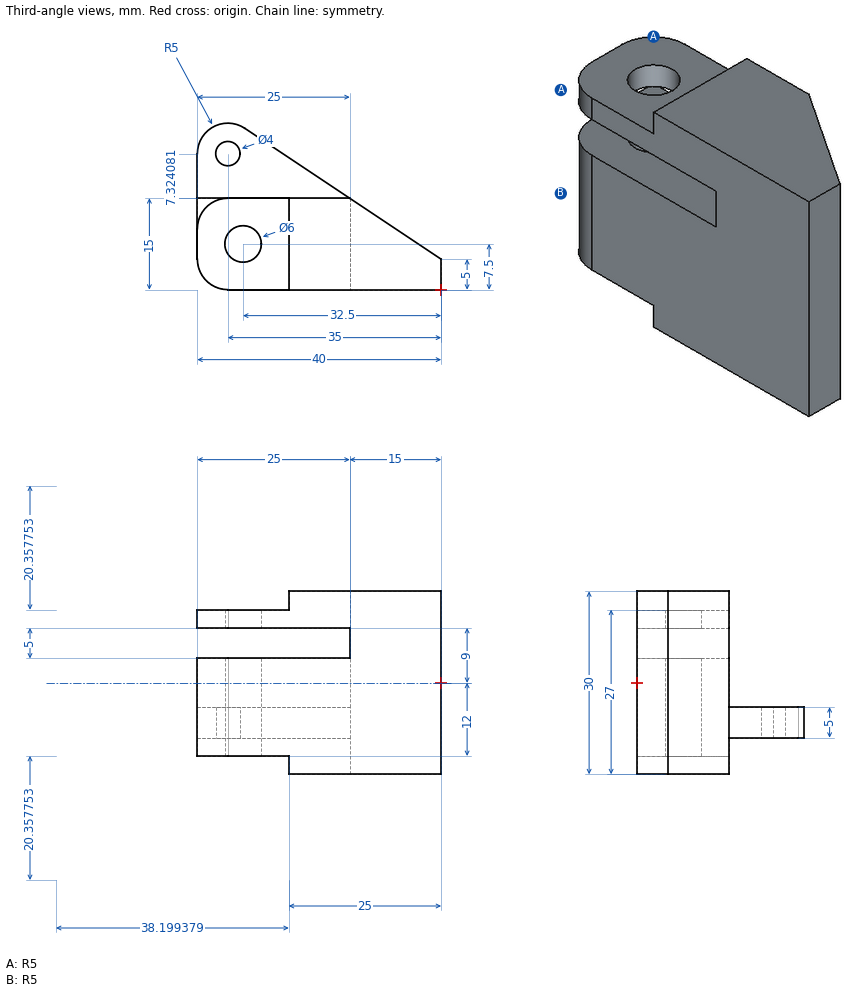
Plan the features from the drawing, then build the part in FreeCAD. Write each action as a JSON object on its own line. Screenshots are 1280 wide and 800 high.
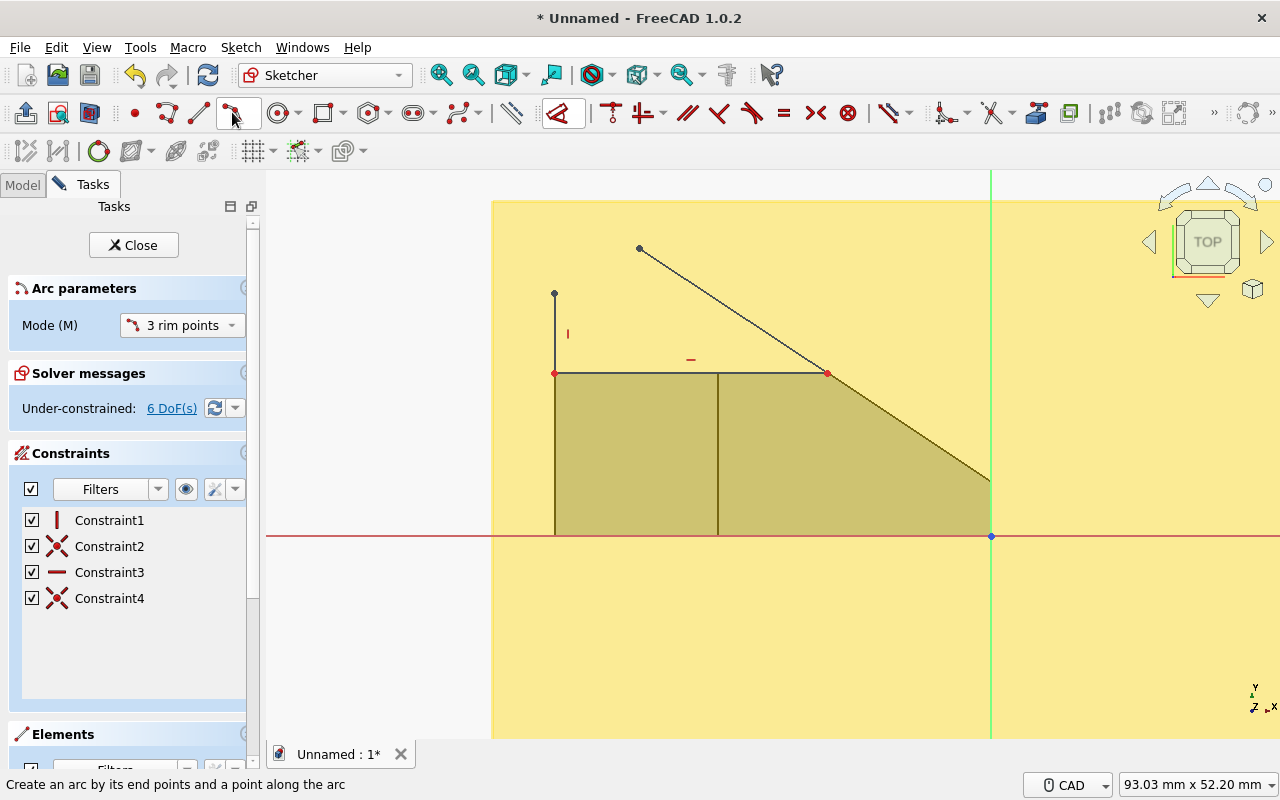
{"action": "left_click", "coordinate": [639, 249]}
{"action": "left_click", "coordinate": [555, 294]}
{"action": "left_click", "coordinate": [584, 245]}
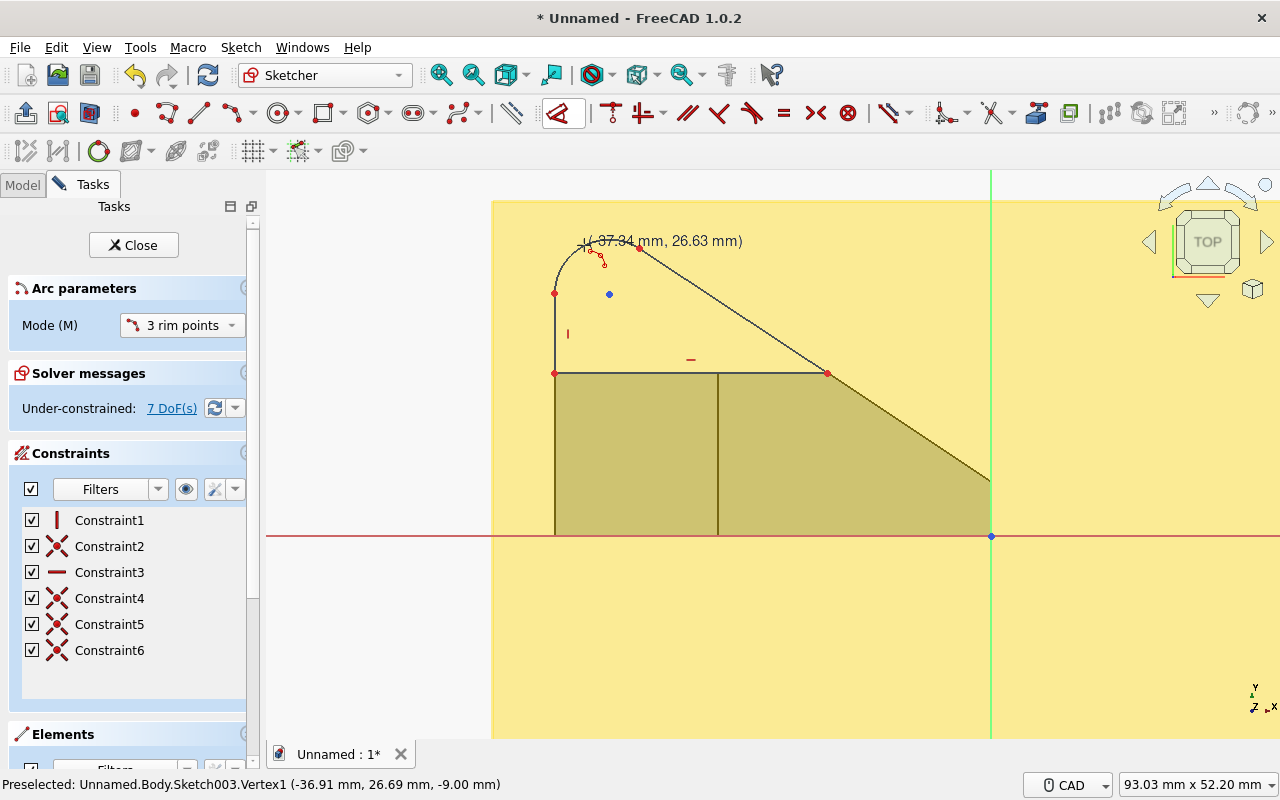
{"action": "key", "text": "g c"}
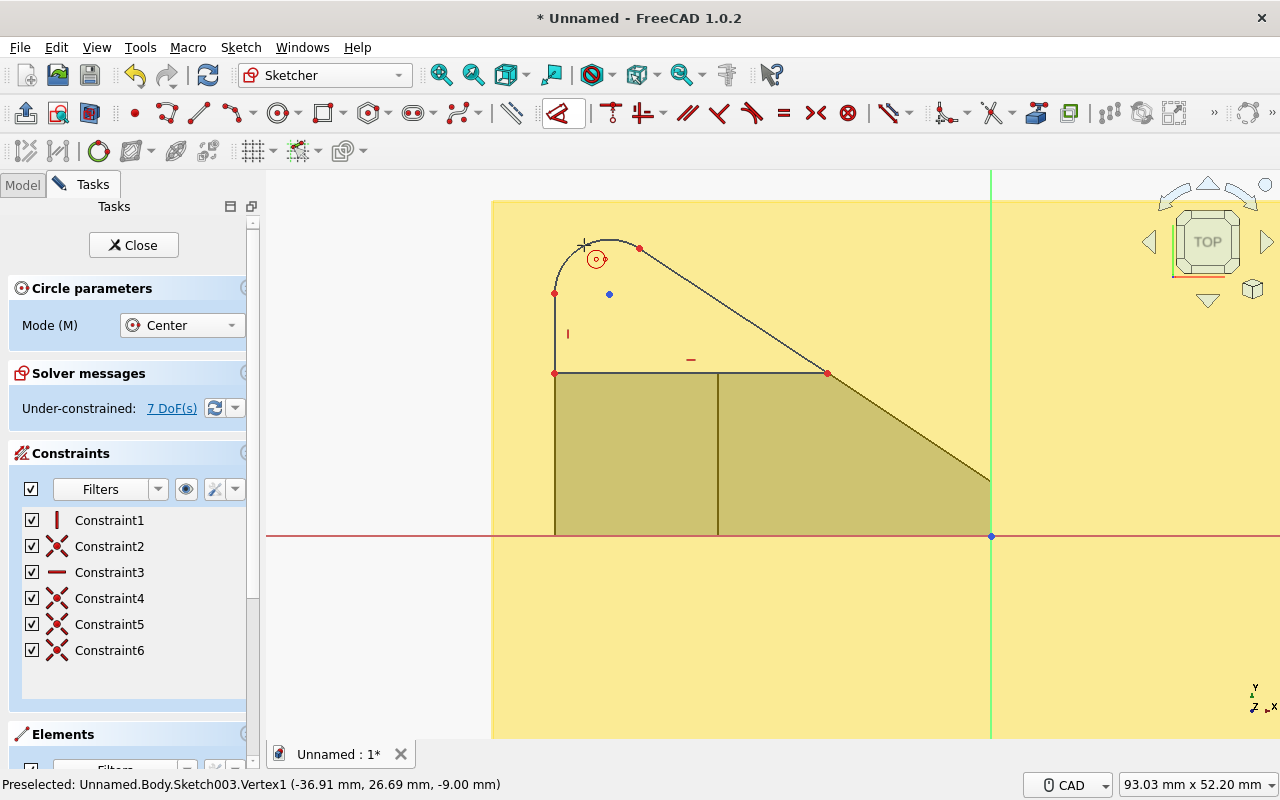
{"action": "left_click", "coordinate": [609, 293]}
{"action": "mouse_move", "coordinate": [625, 278]}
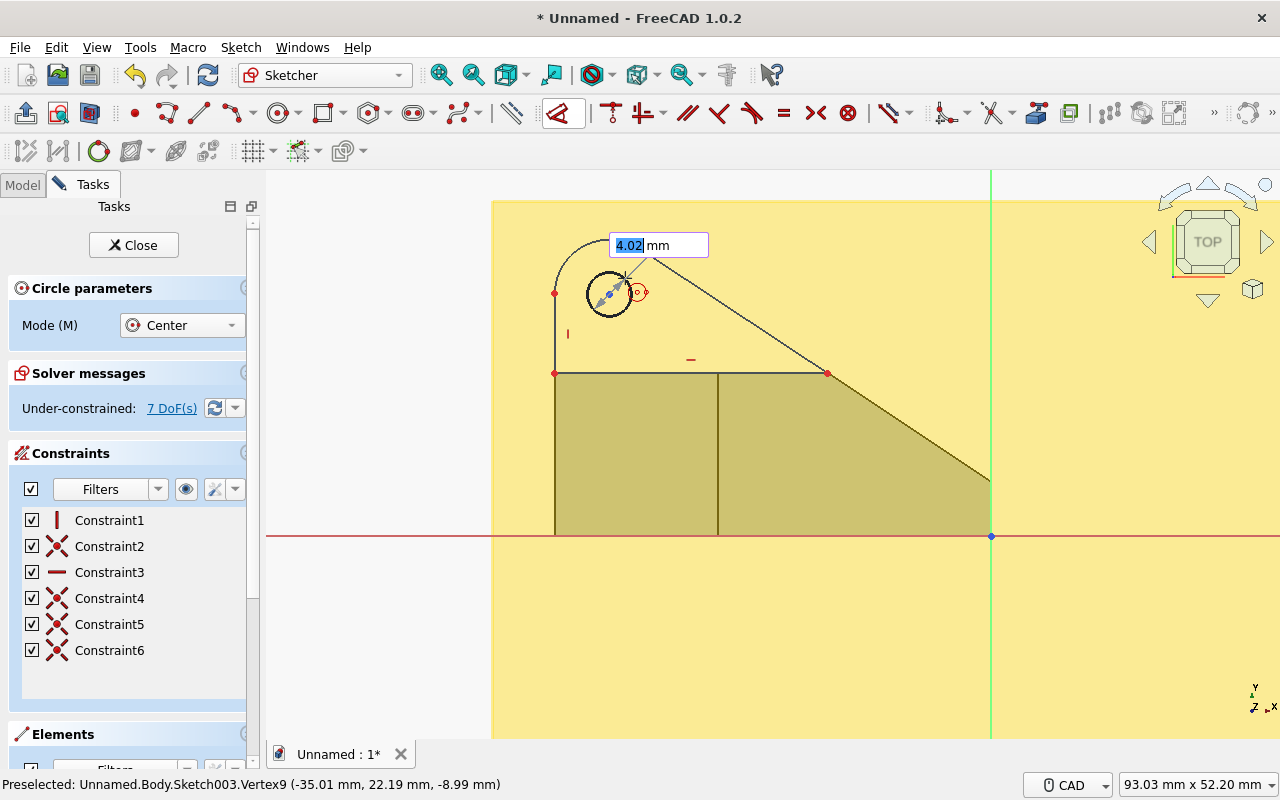
{"action": "type", "text": "4"}
{"action": "key", "text": "Return"}
{"action": "key", "text": "Escape"}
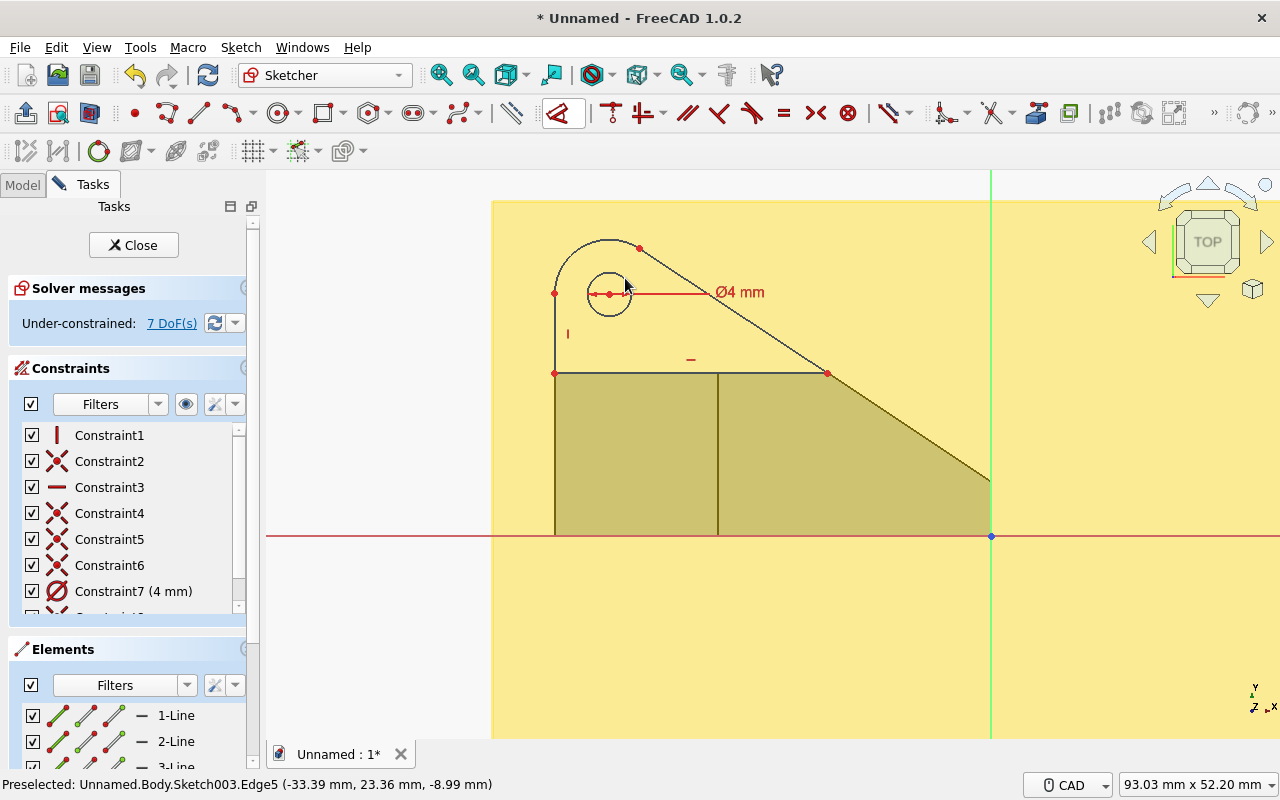
{"action": "left_click", "coordinate": [555, 317]}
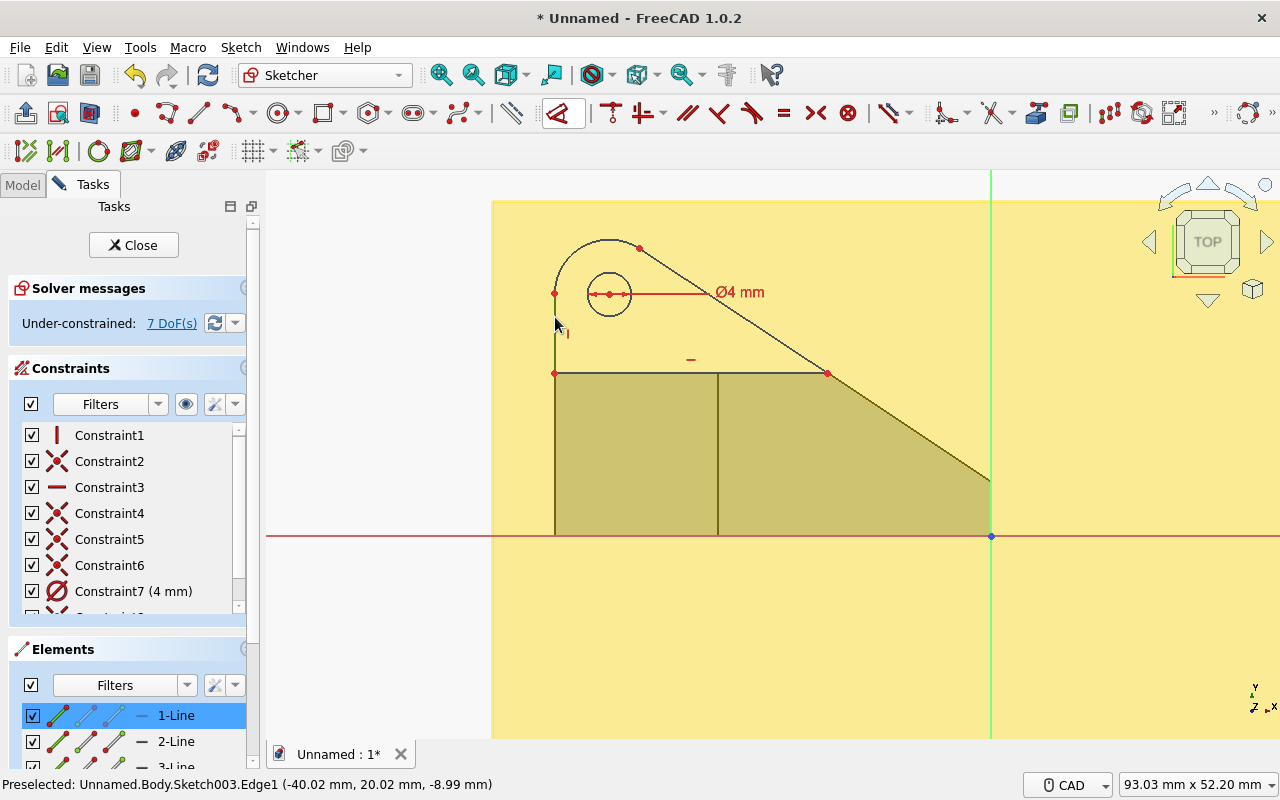
{"action": "left_click", "coordinate": [606, 240]}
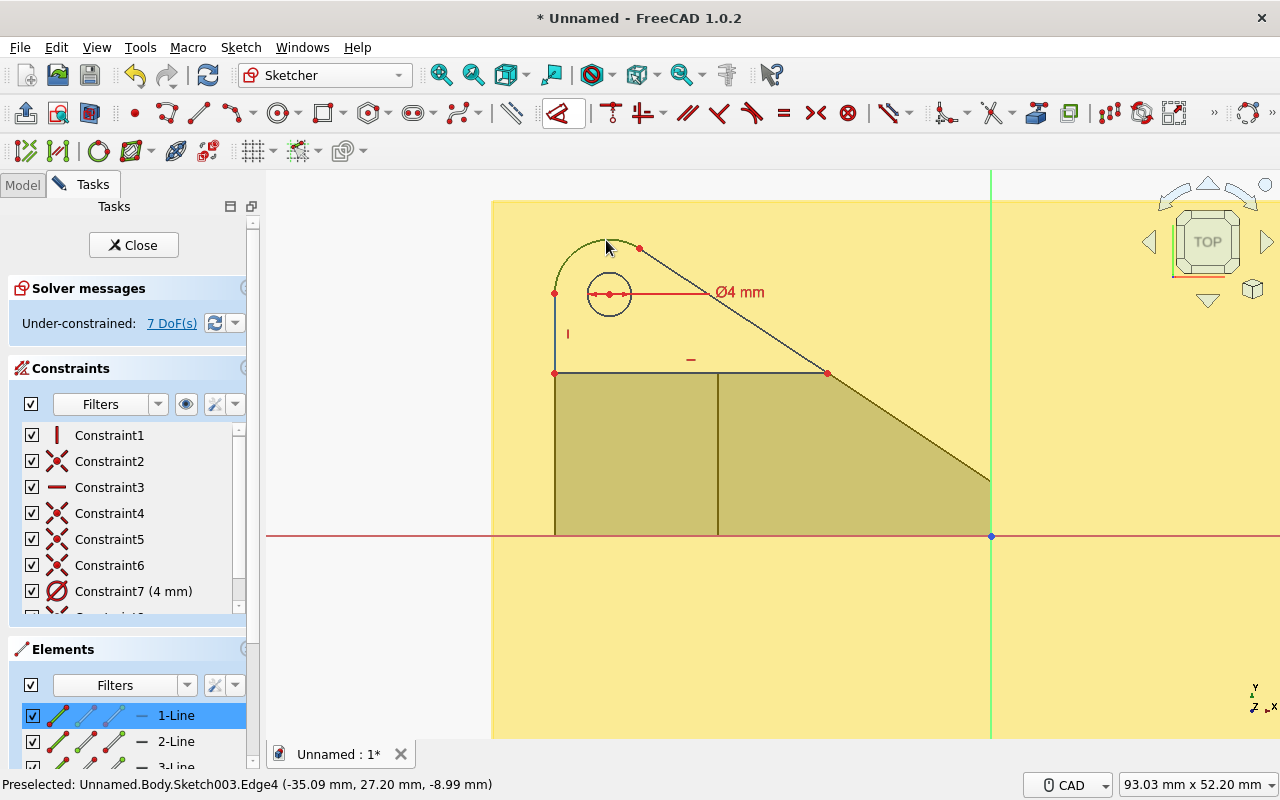
{"action": "key", "text": "t"}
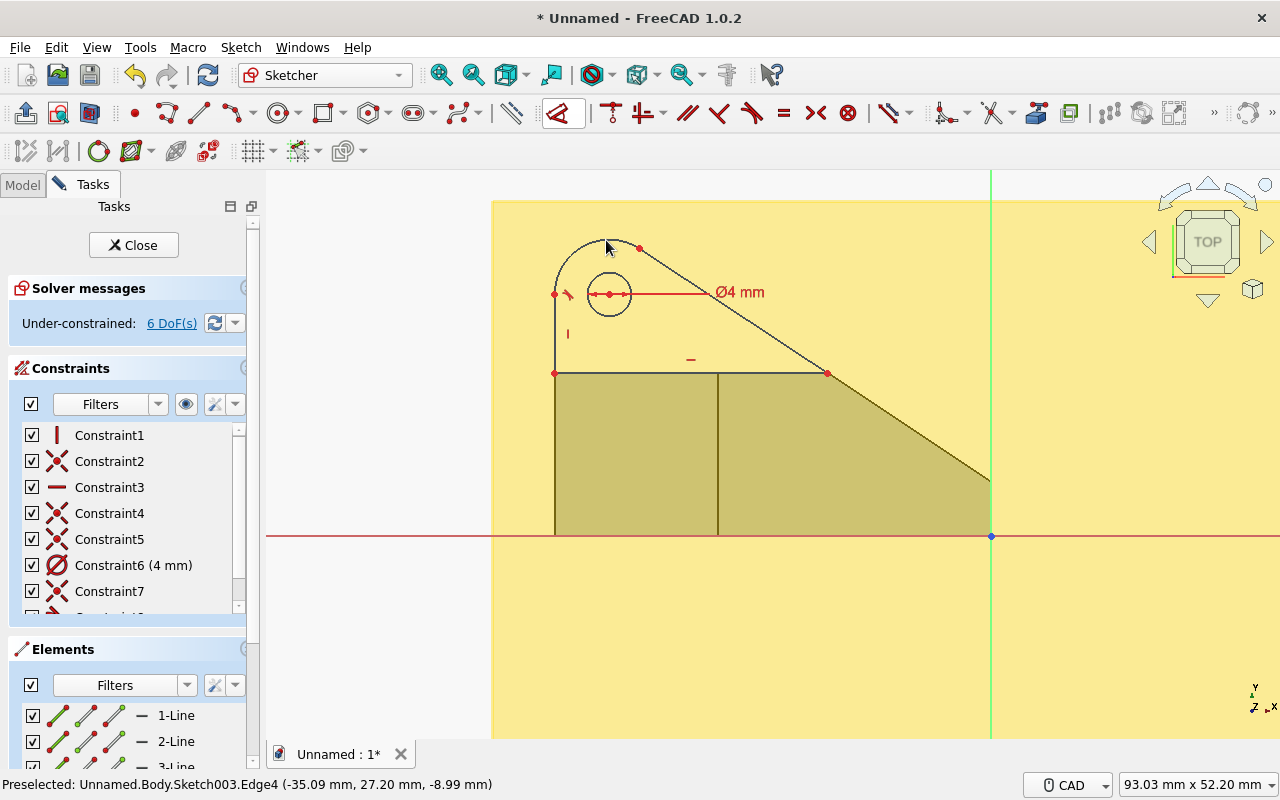
{"action": "left_click", "coordinate": [771, 336]}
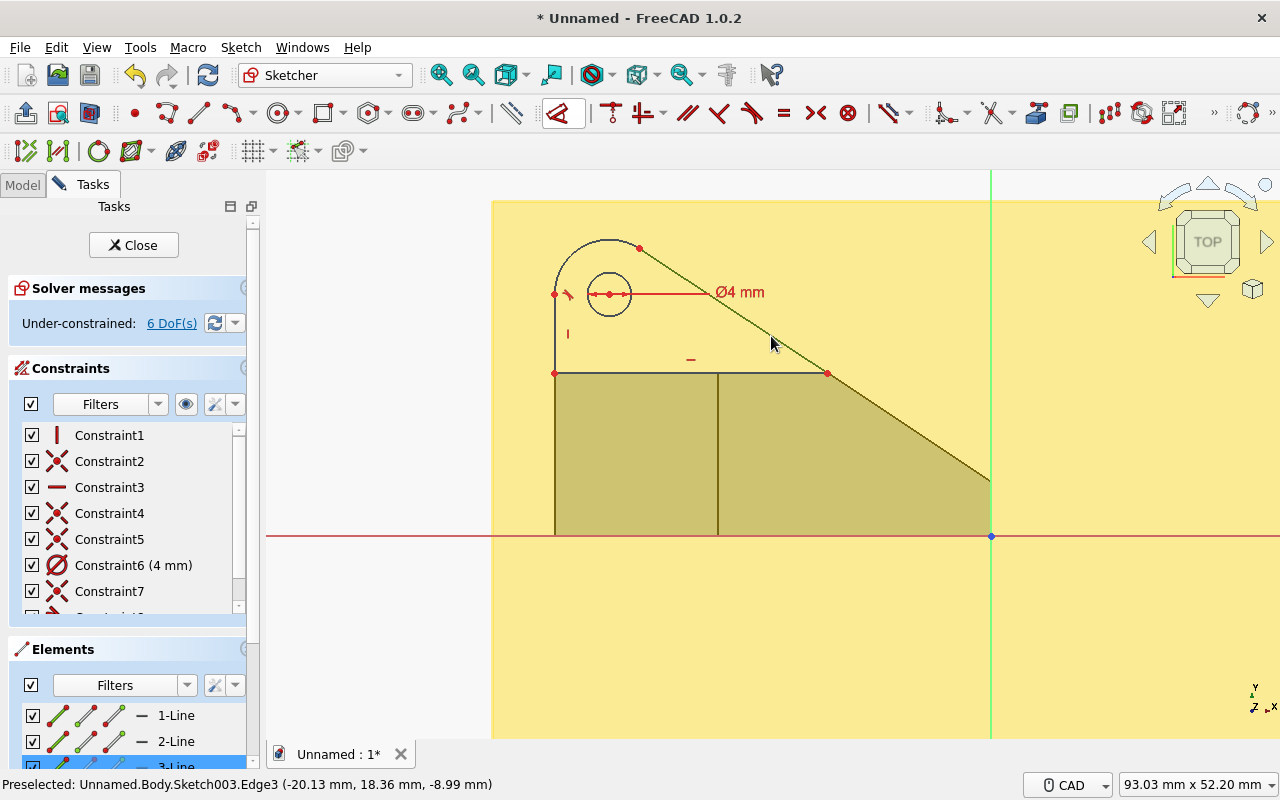
{"action": "left_click", "coordinate": [606, 240]}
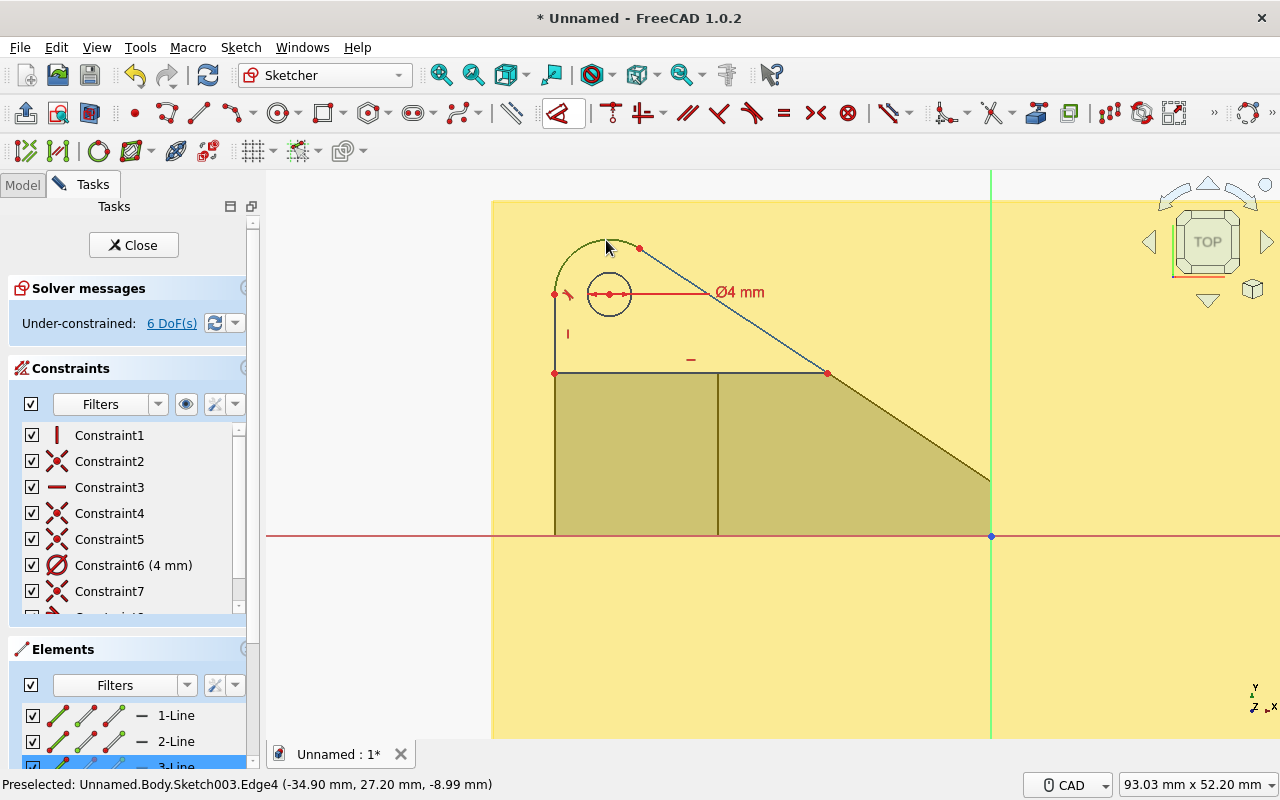
{"action": "left_click", "coordinate": [752, 114]}